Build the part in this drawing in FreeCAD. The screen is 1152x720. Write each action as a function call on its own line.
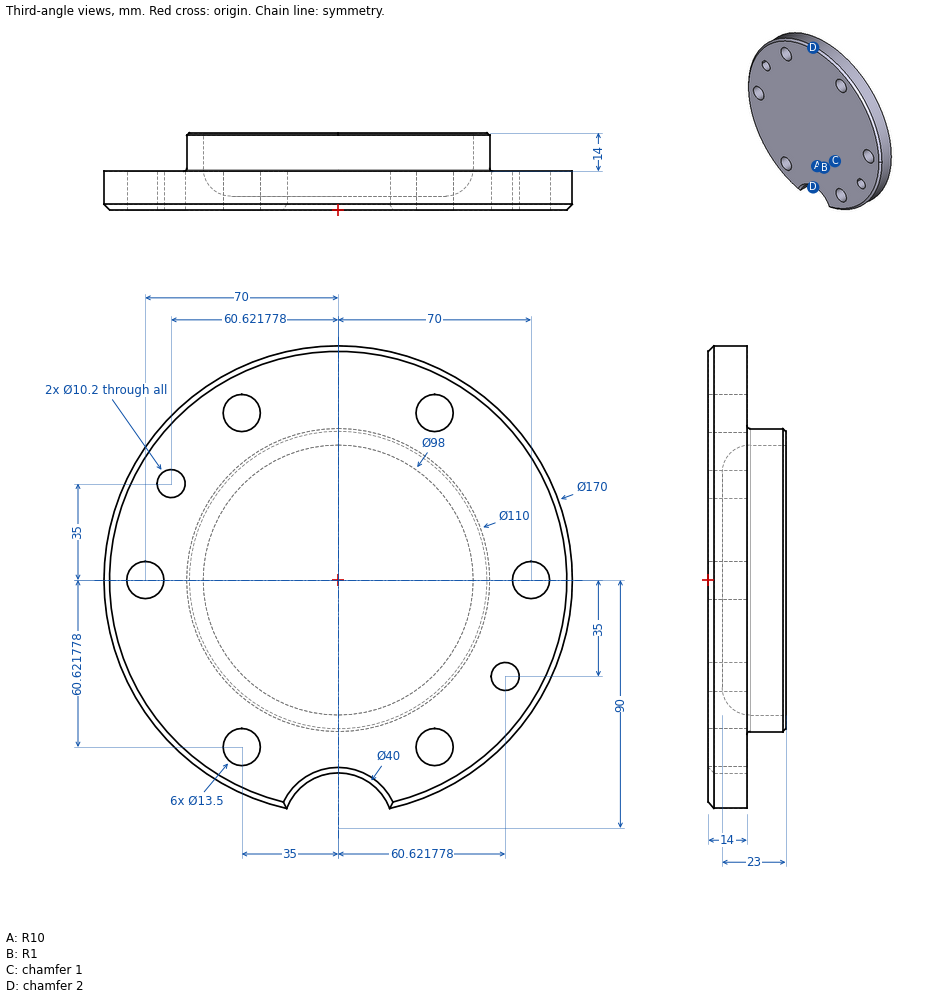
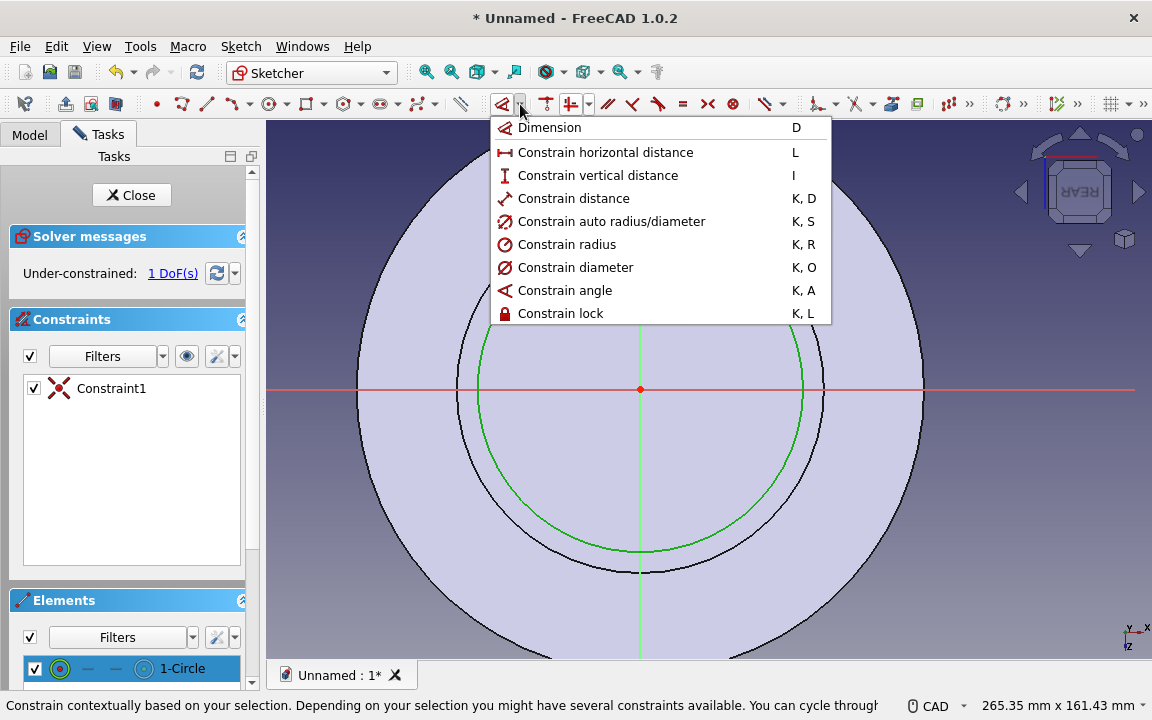
click(661, 268)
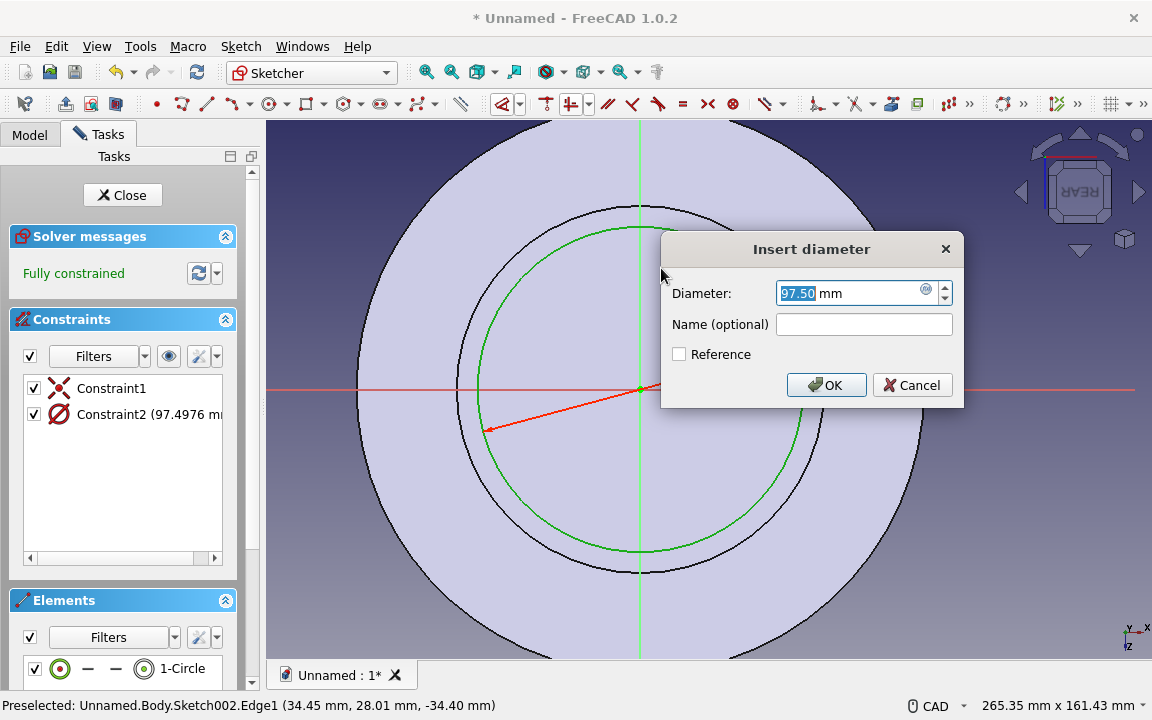
text(98)
key(Return)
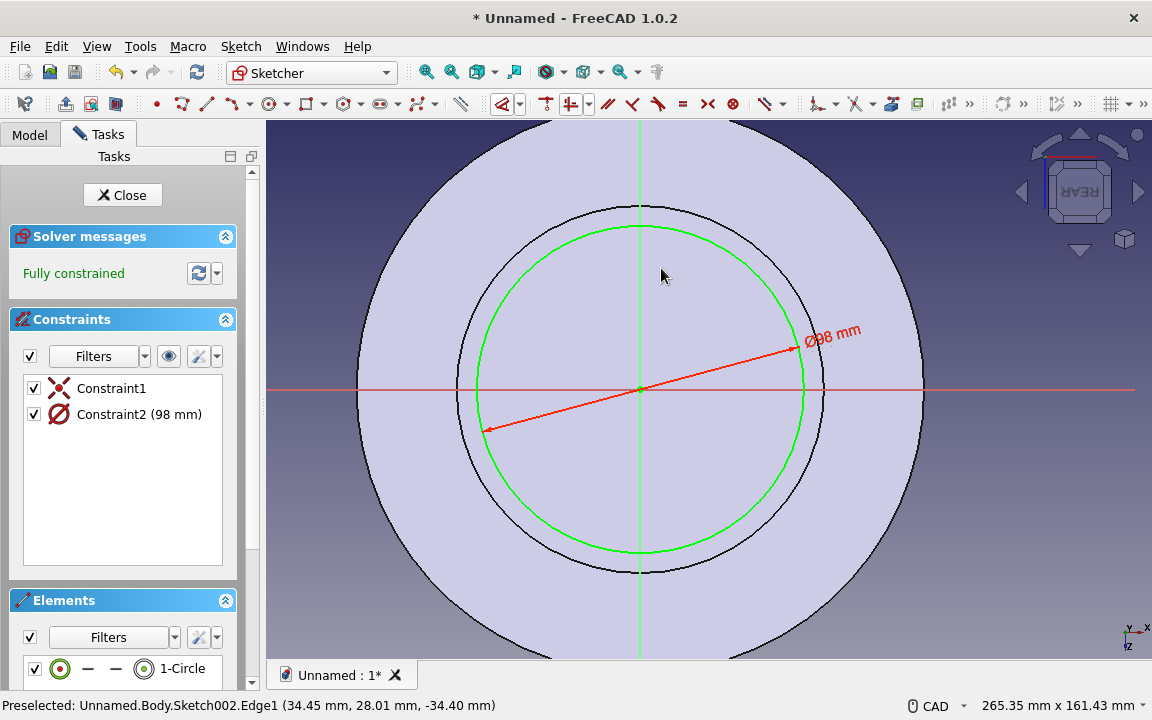
click(123, 195)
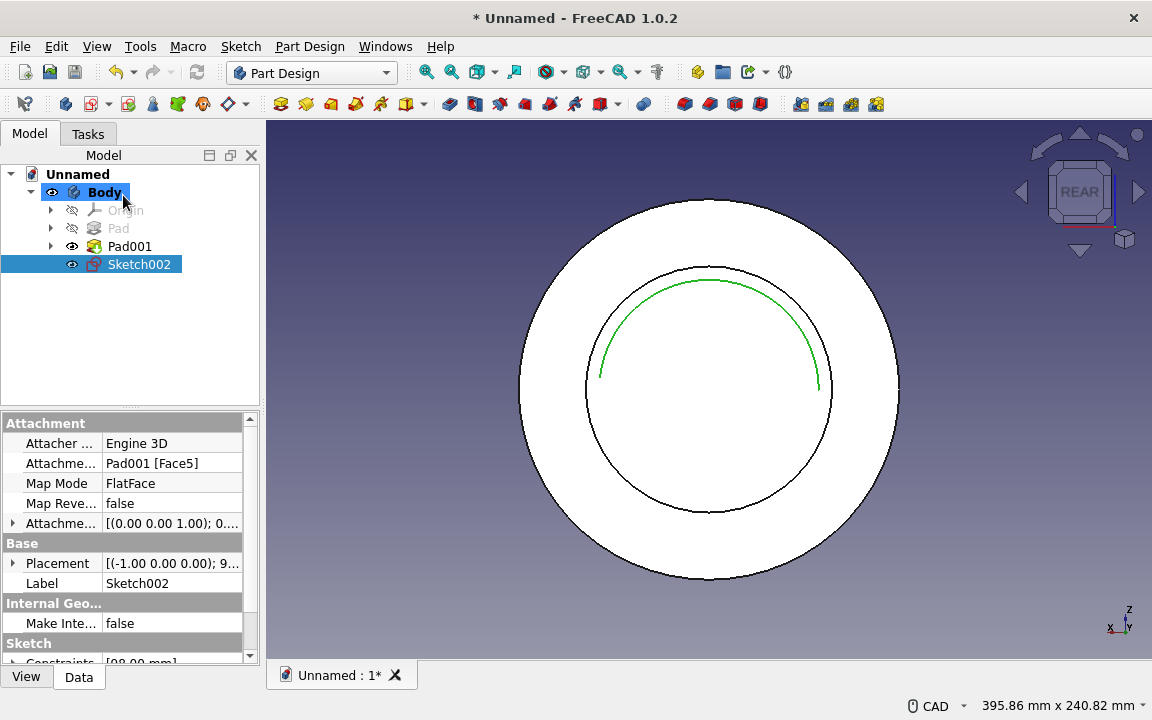
click(450, 104)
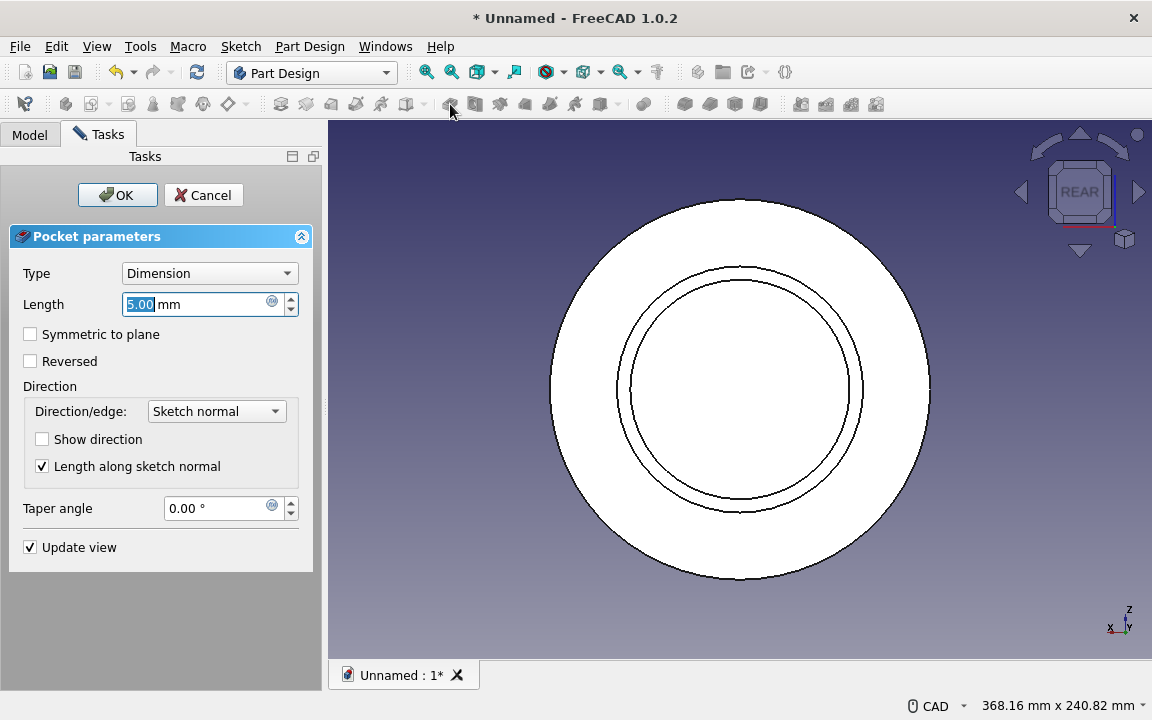
text(23)
key(Tab)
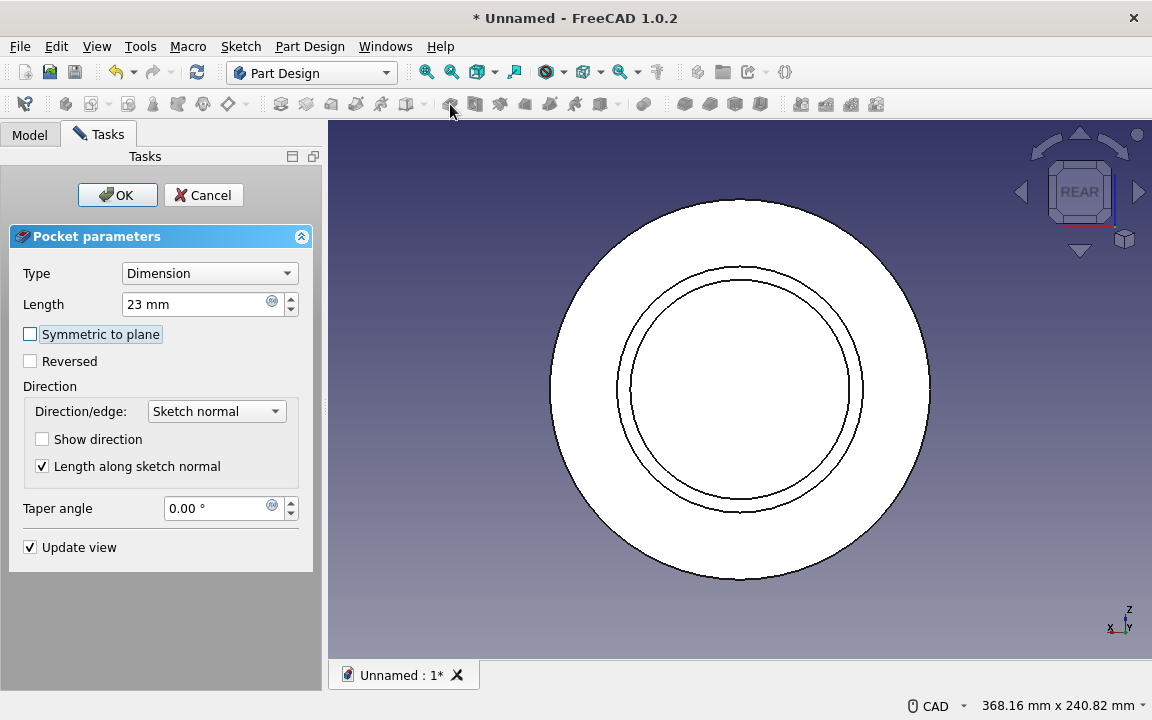
click(118, 195)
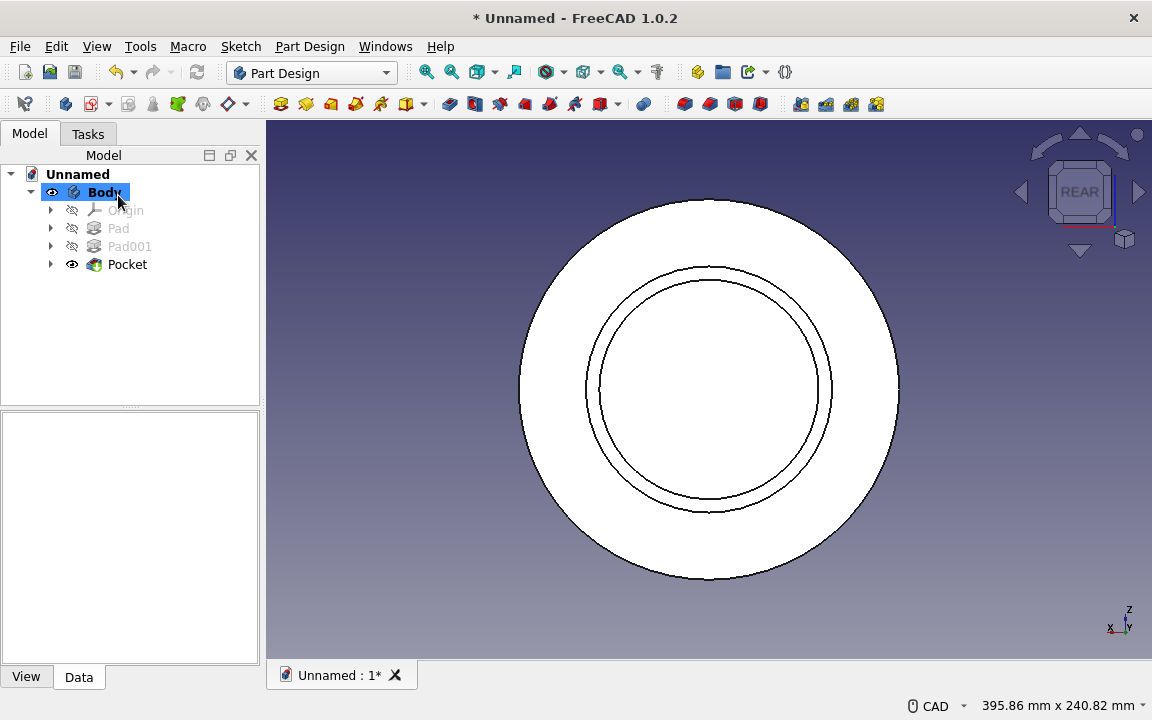
key(0)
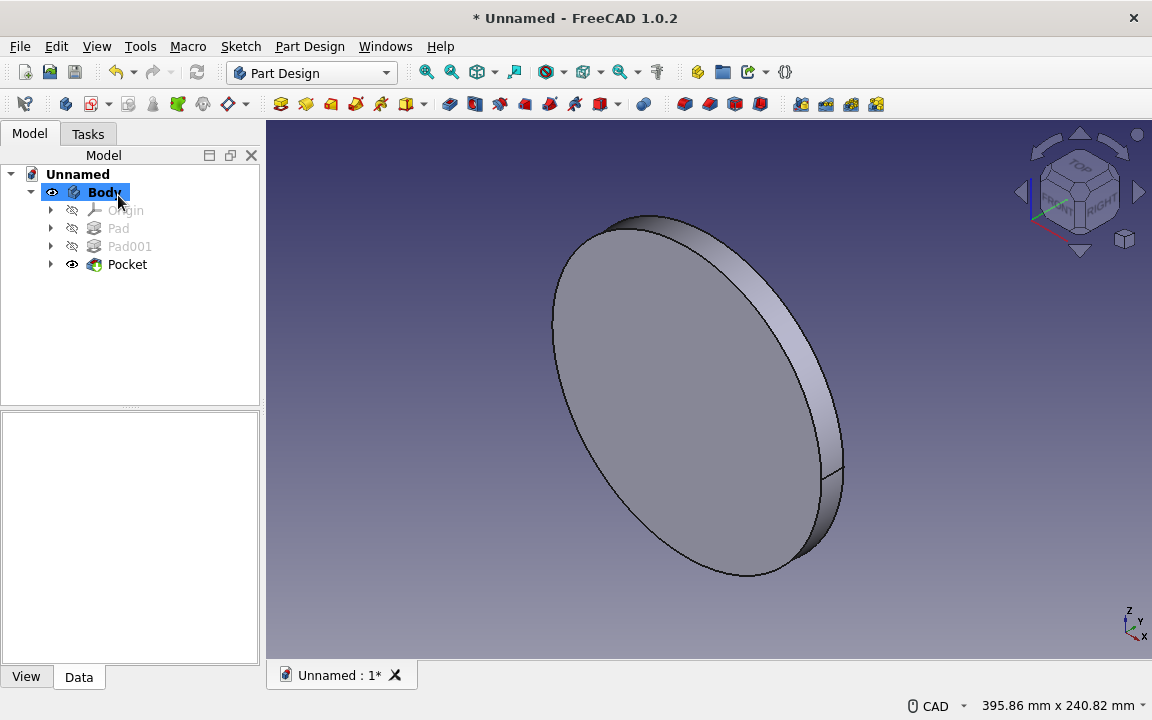
key(2)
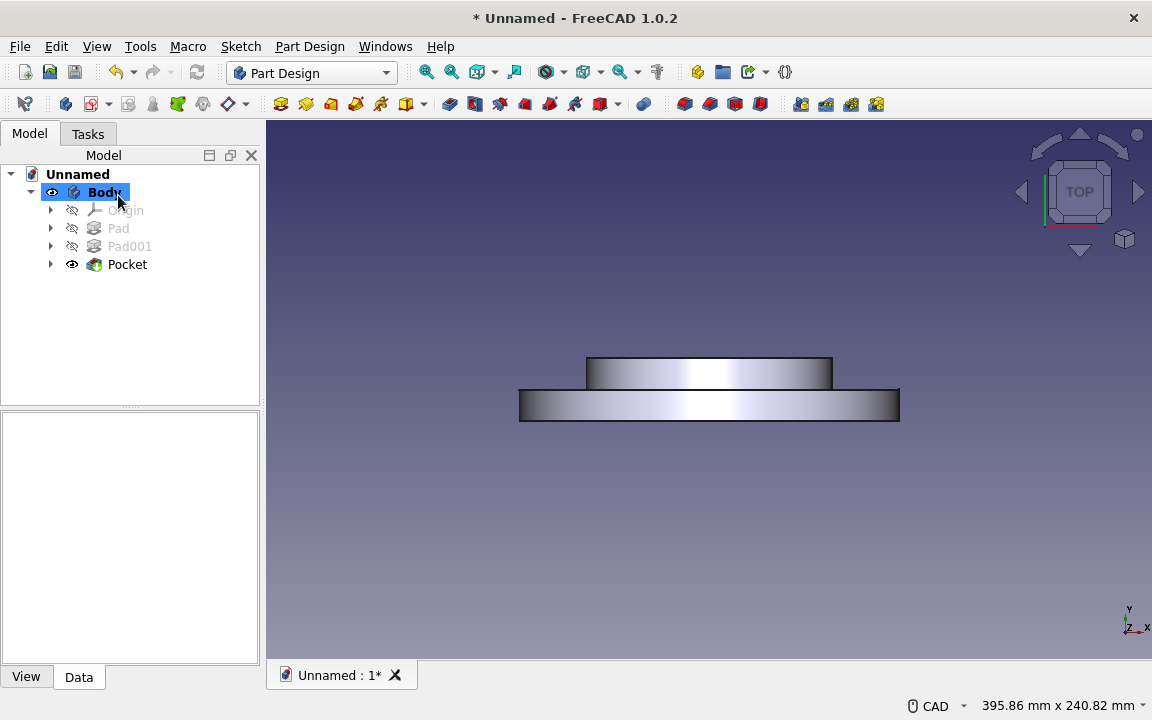
click(427, 72)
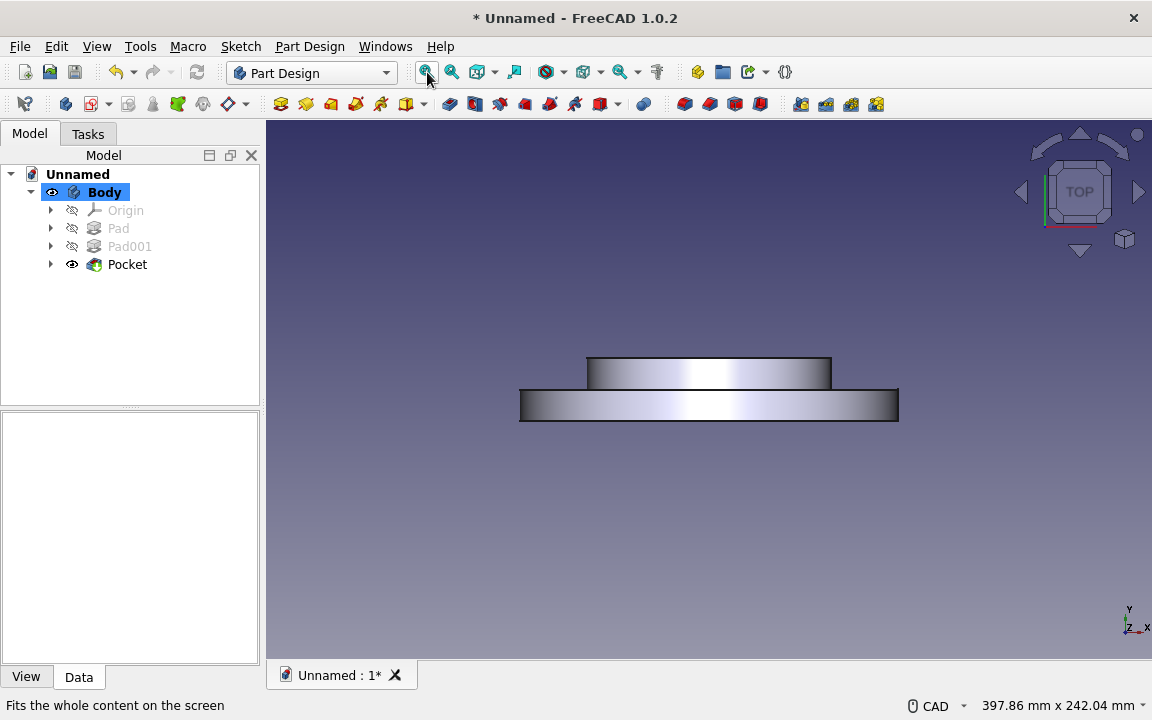
key(1)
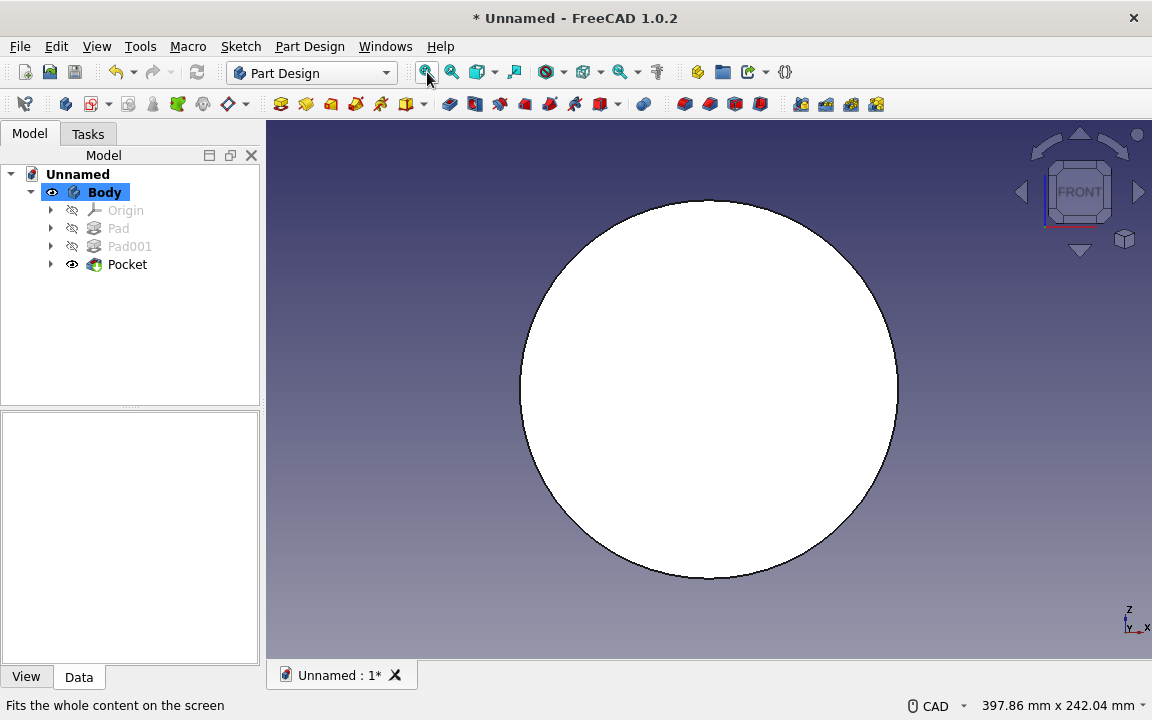
key(3)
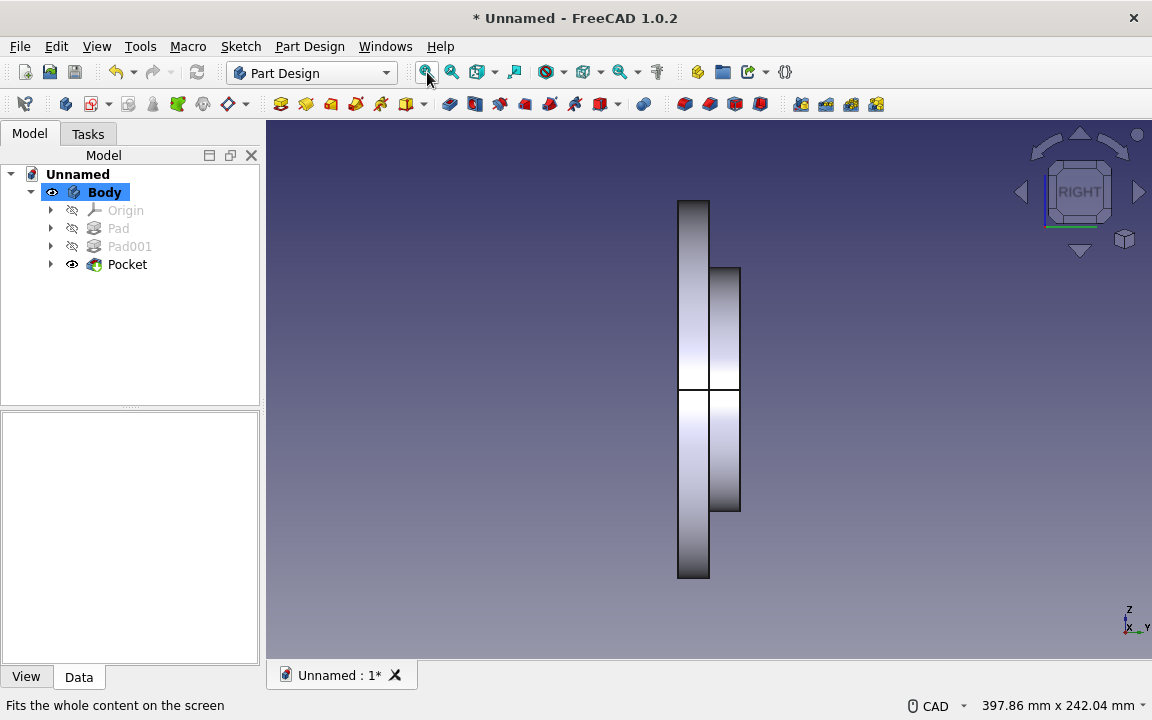
key(5)